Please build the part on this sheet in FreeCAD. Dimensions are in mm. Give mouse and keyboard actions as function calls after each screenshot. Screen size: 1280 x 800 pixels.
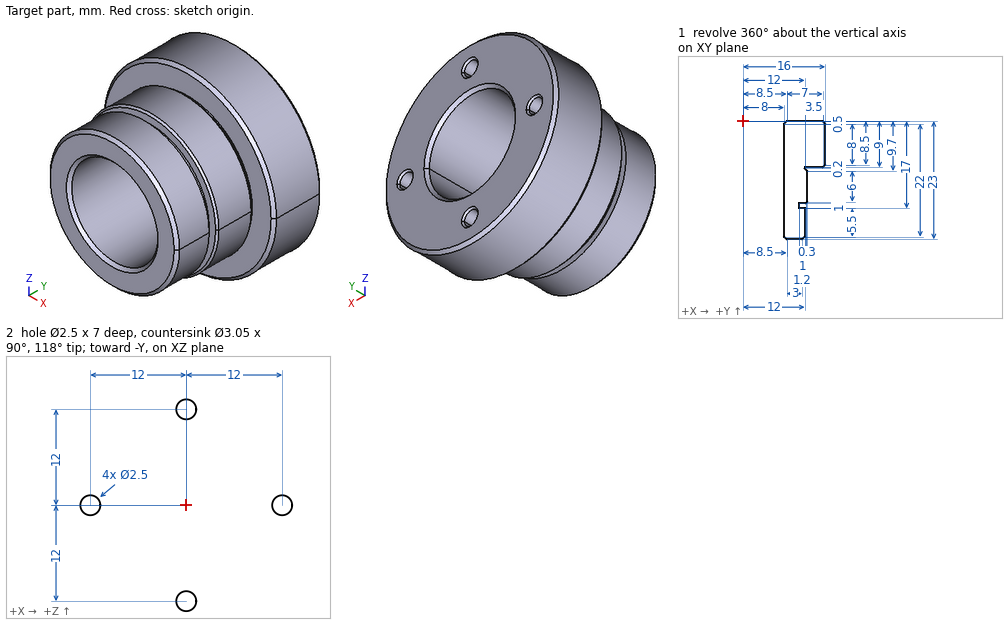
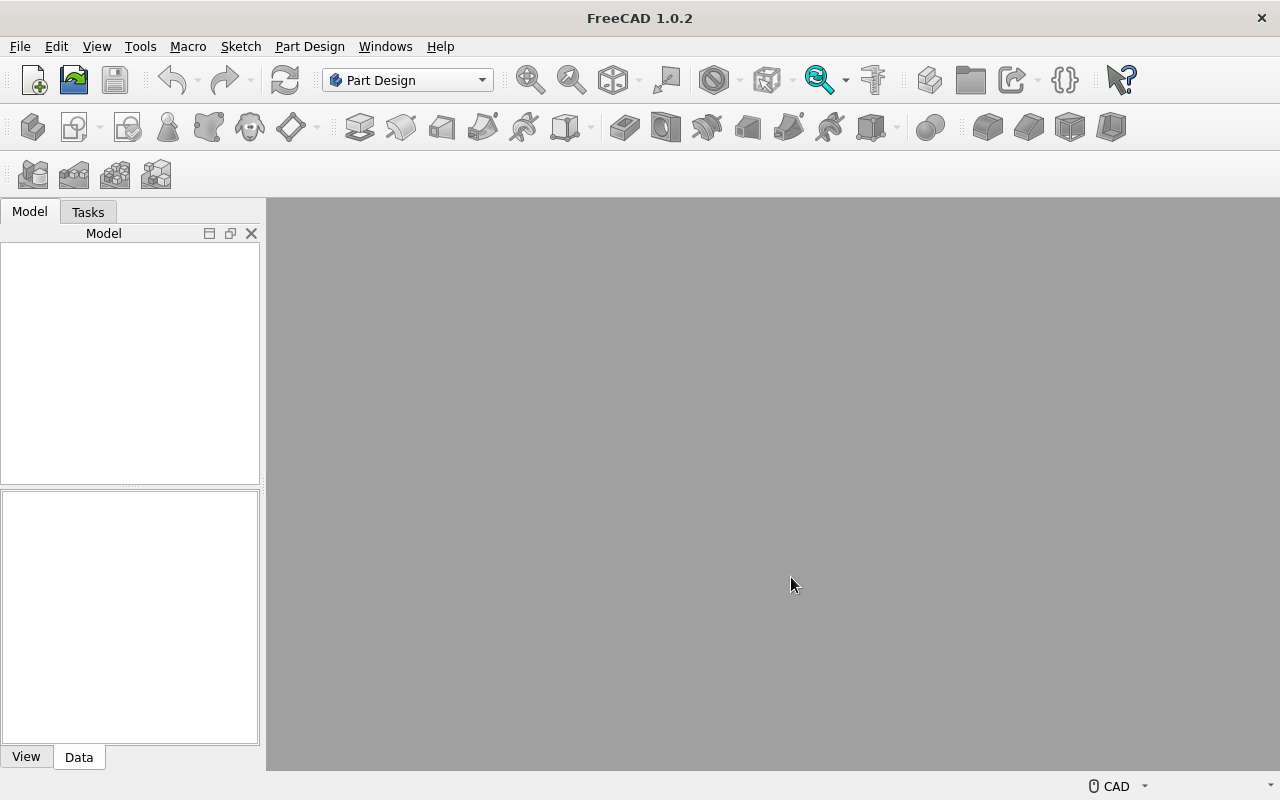
click(33, 80)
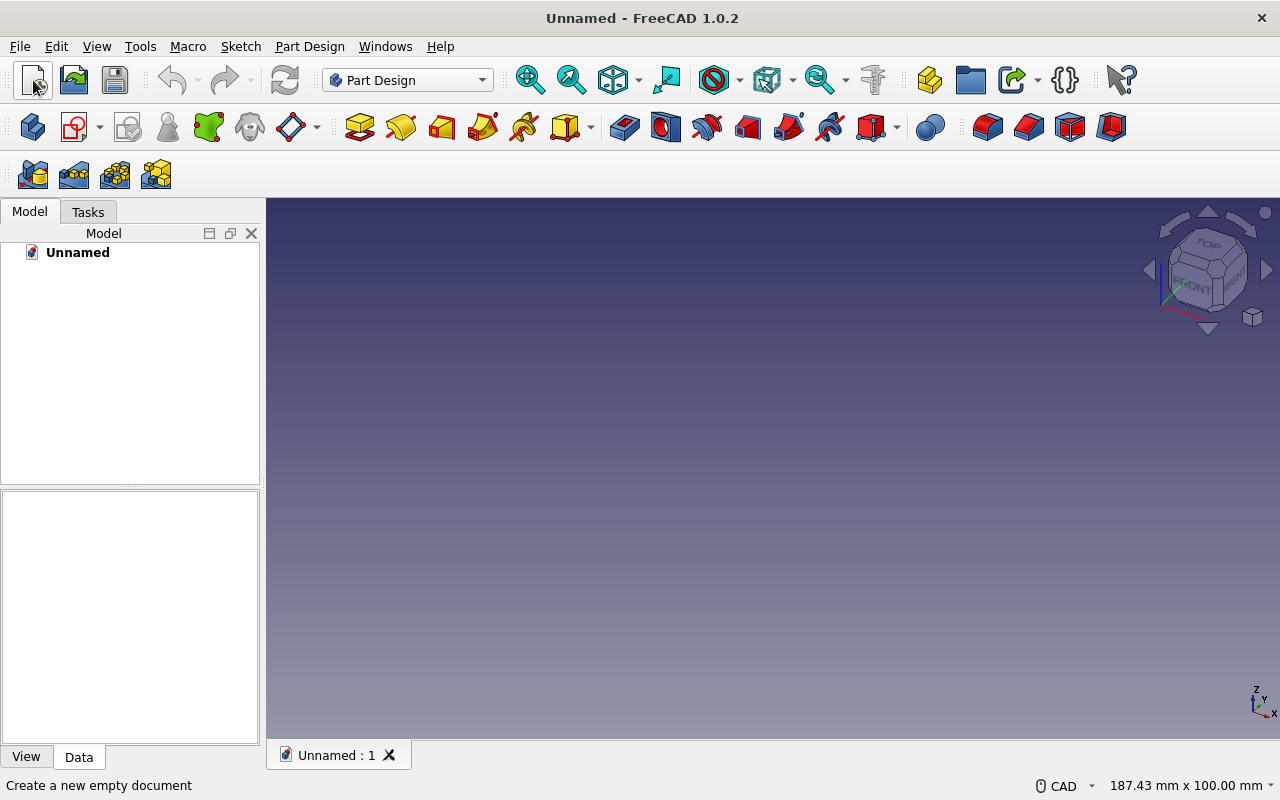
click(74, 128)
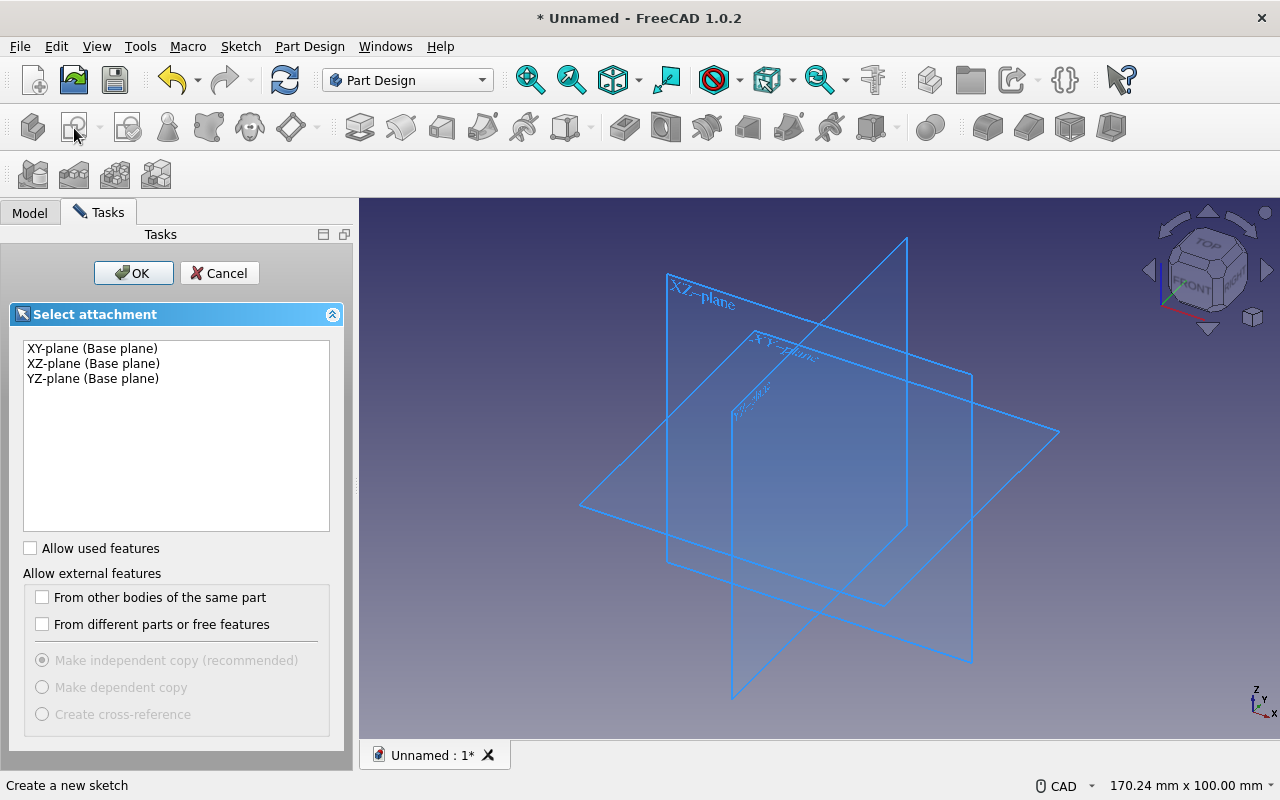
click(84, 348)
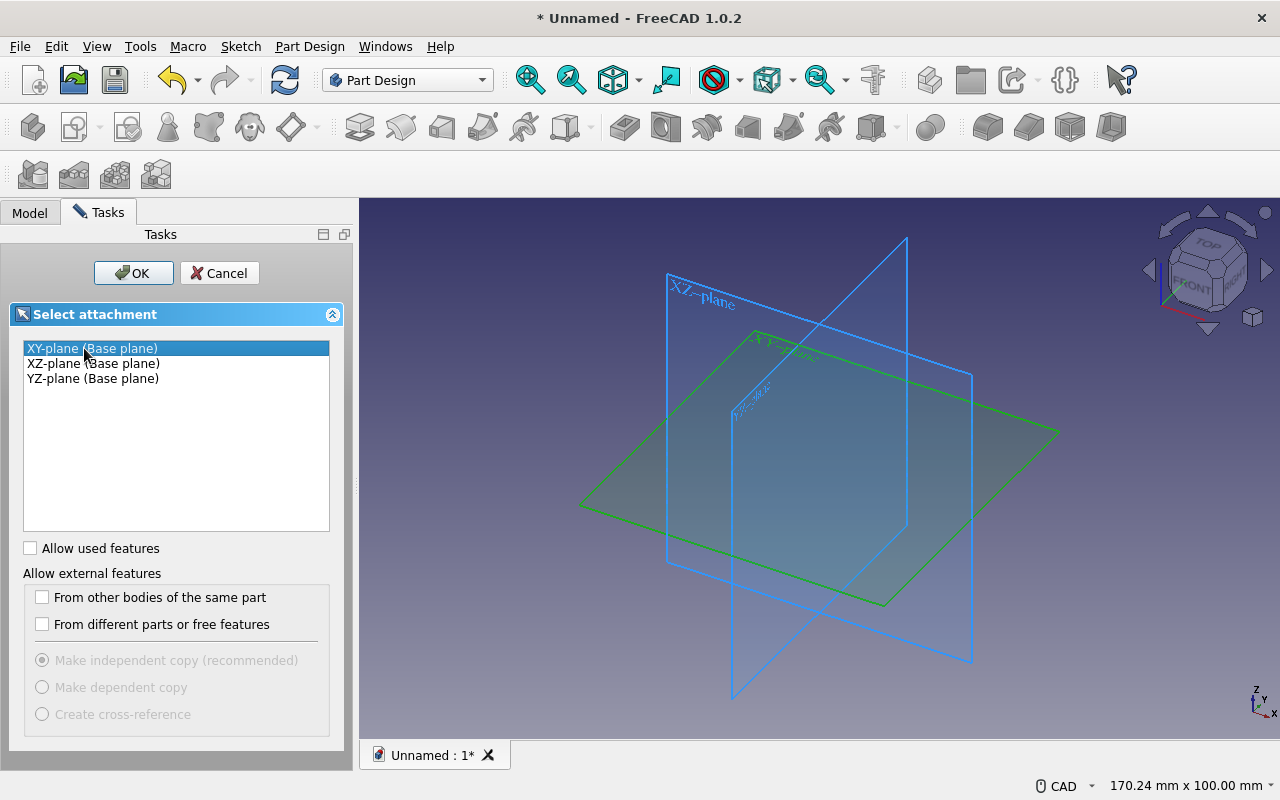
click(134, 273)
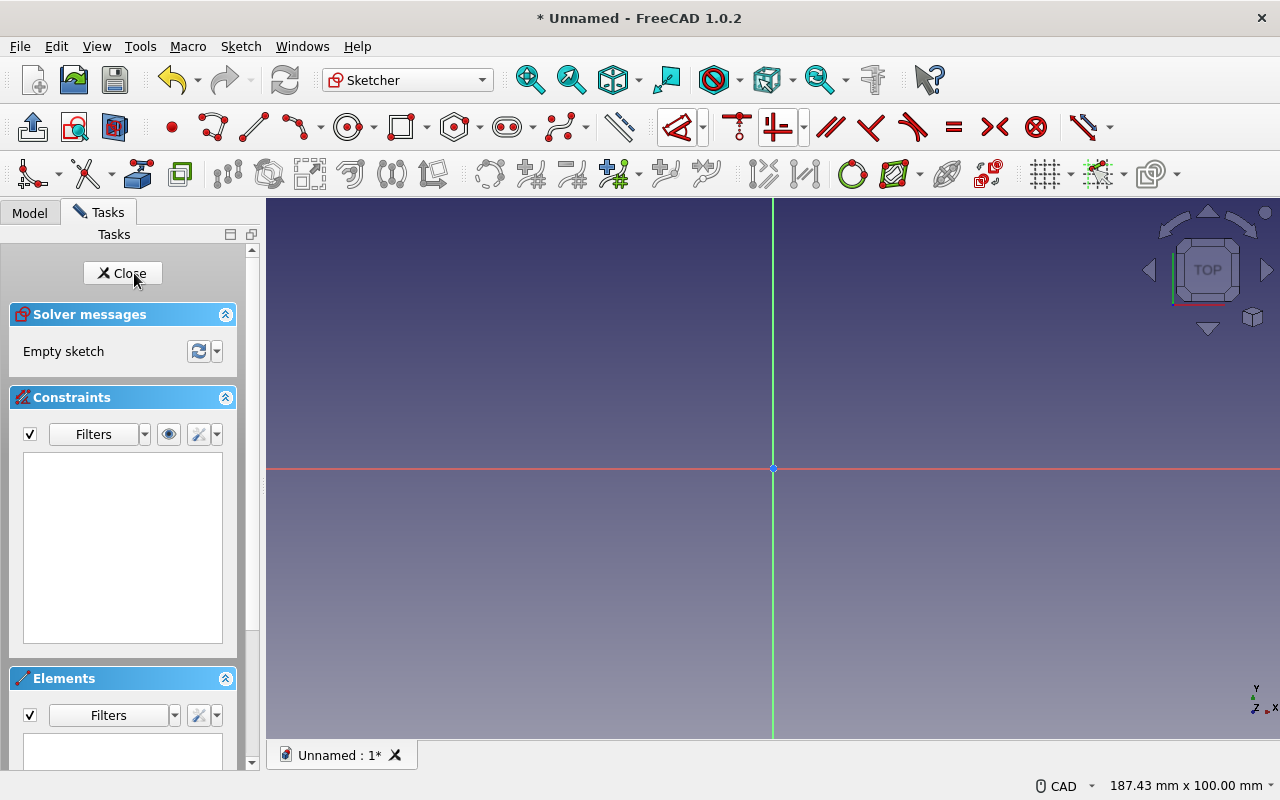
scroll(881, 567, up, 5)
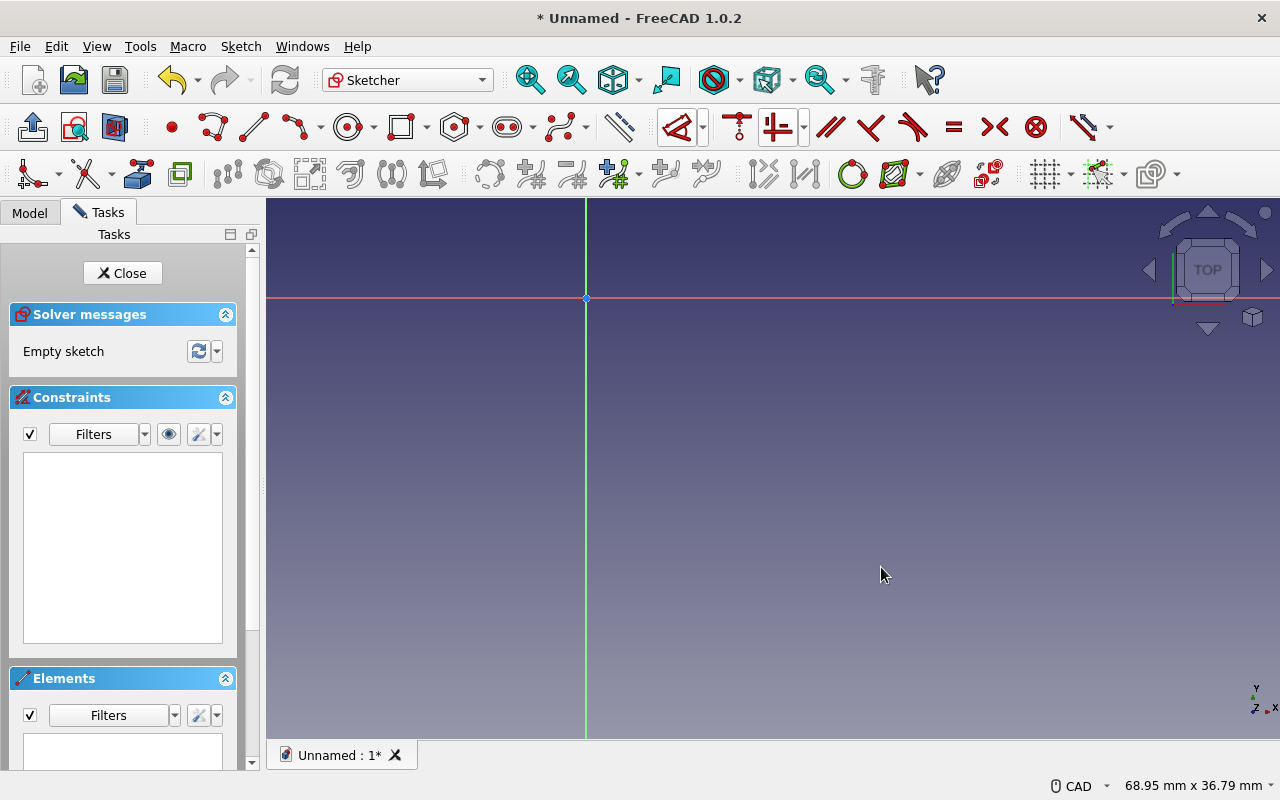
click(213, 128)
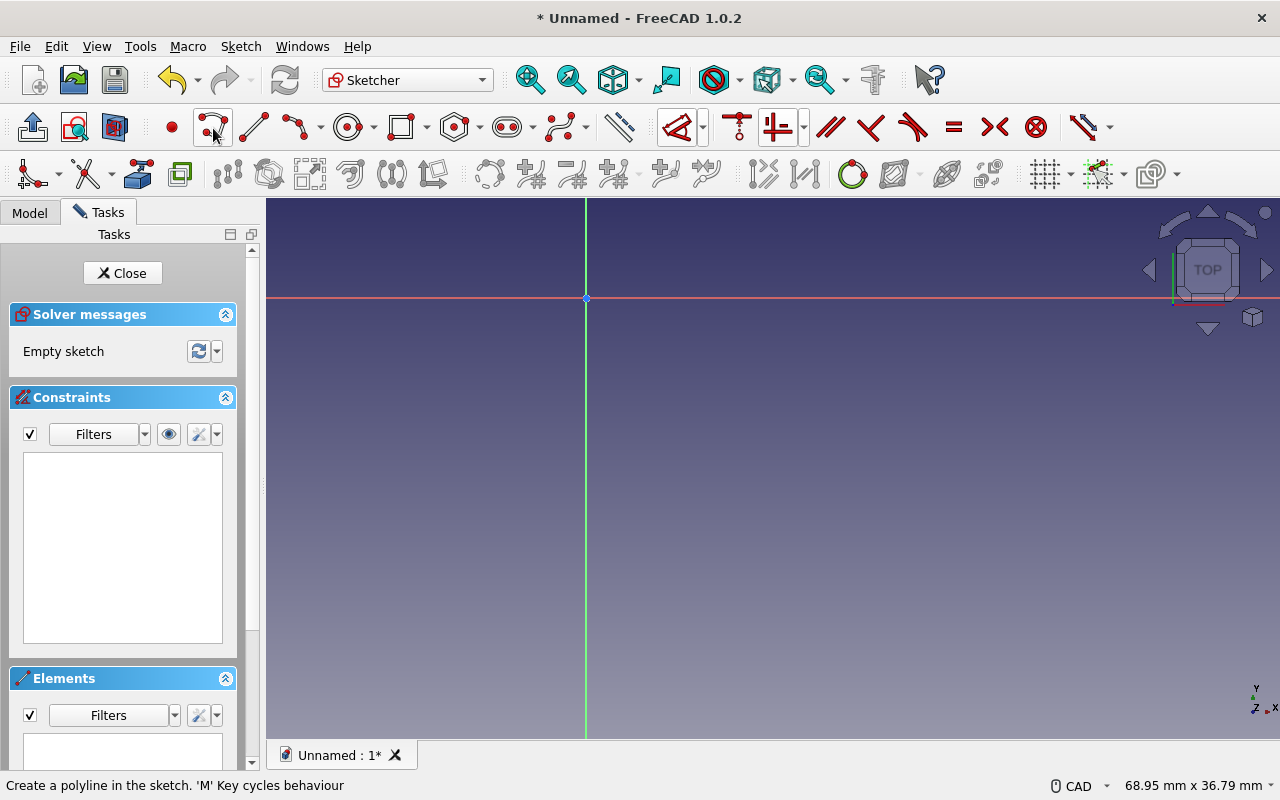
scroll(704, 305, up, 4)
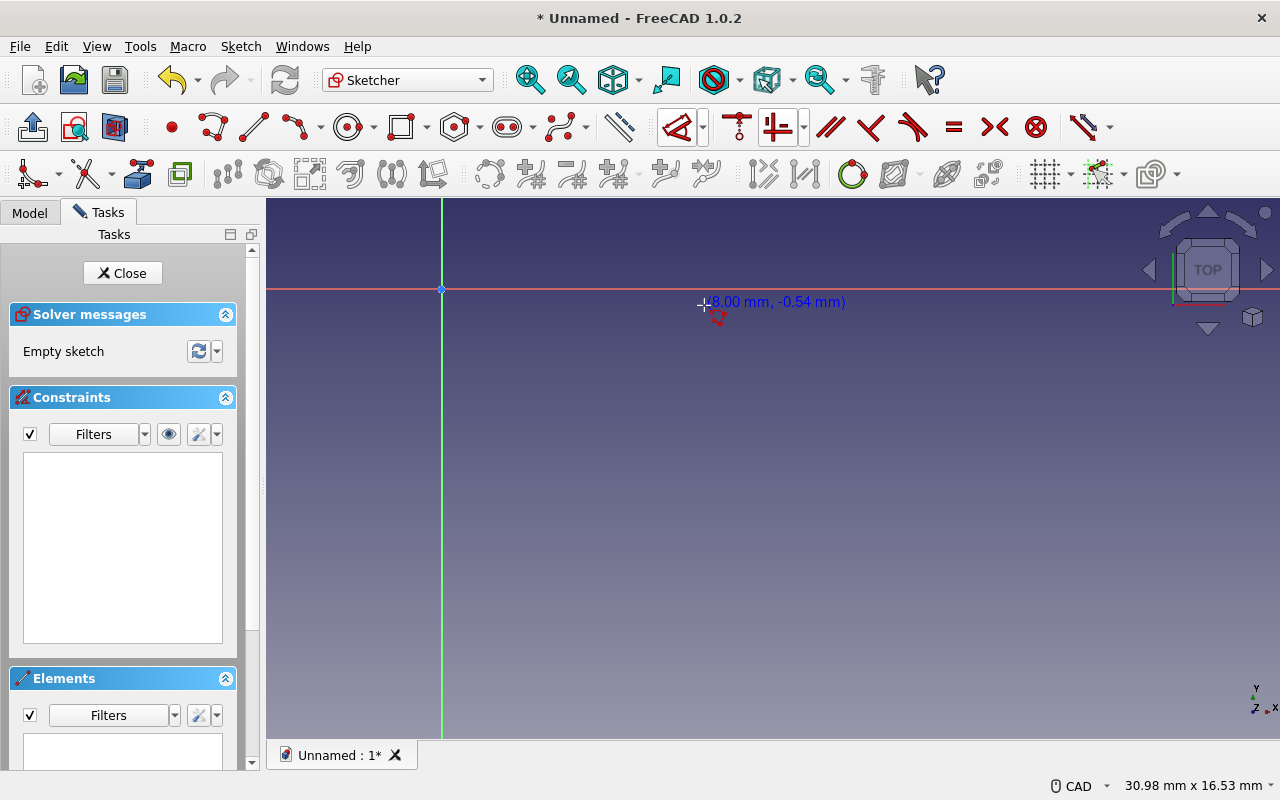
click(704, 306)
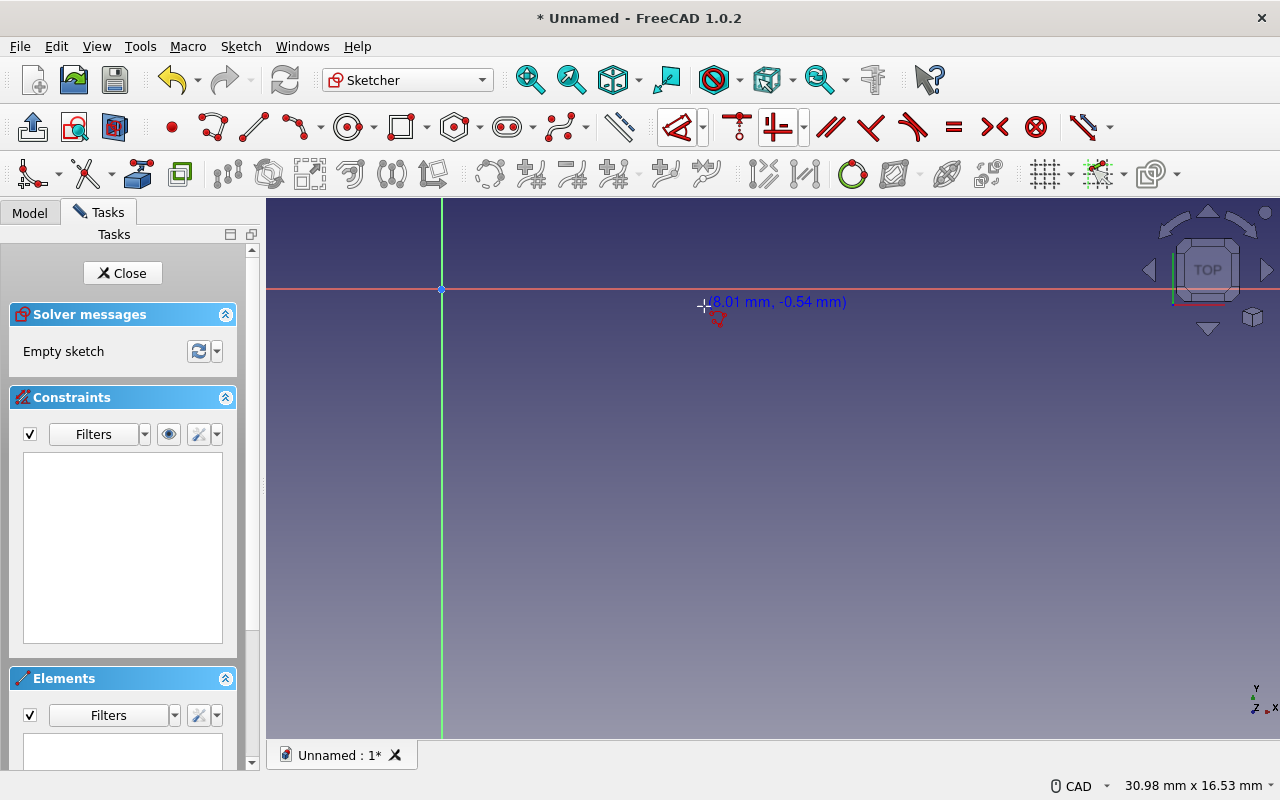
scroll(705, 308, down, 4)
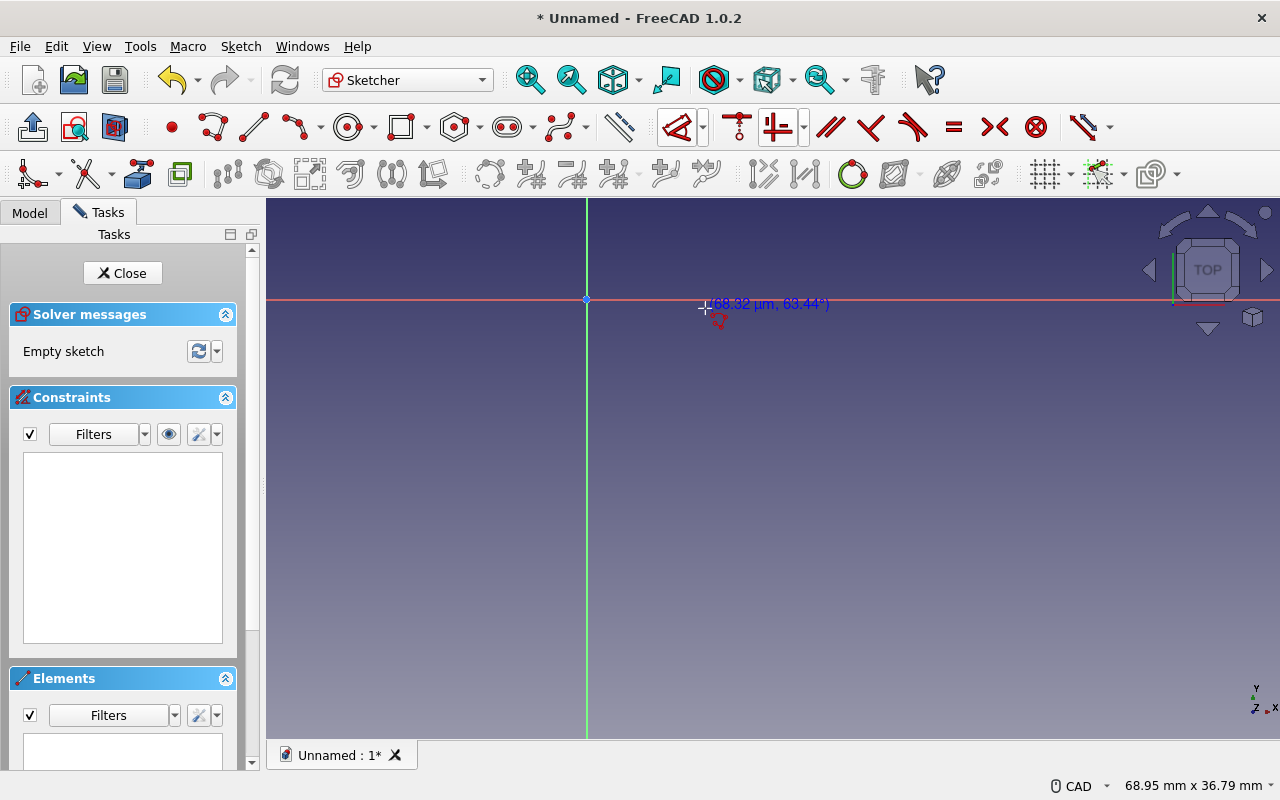
click(705, 631)